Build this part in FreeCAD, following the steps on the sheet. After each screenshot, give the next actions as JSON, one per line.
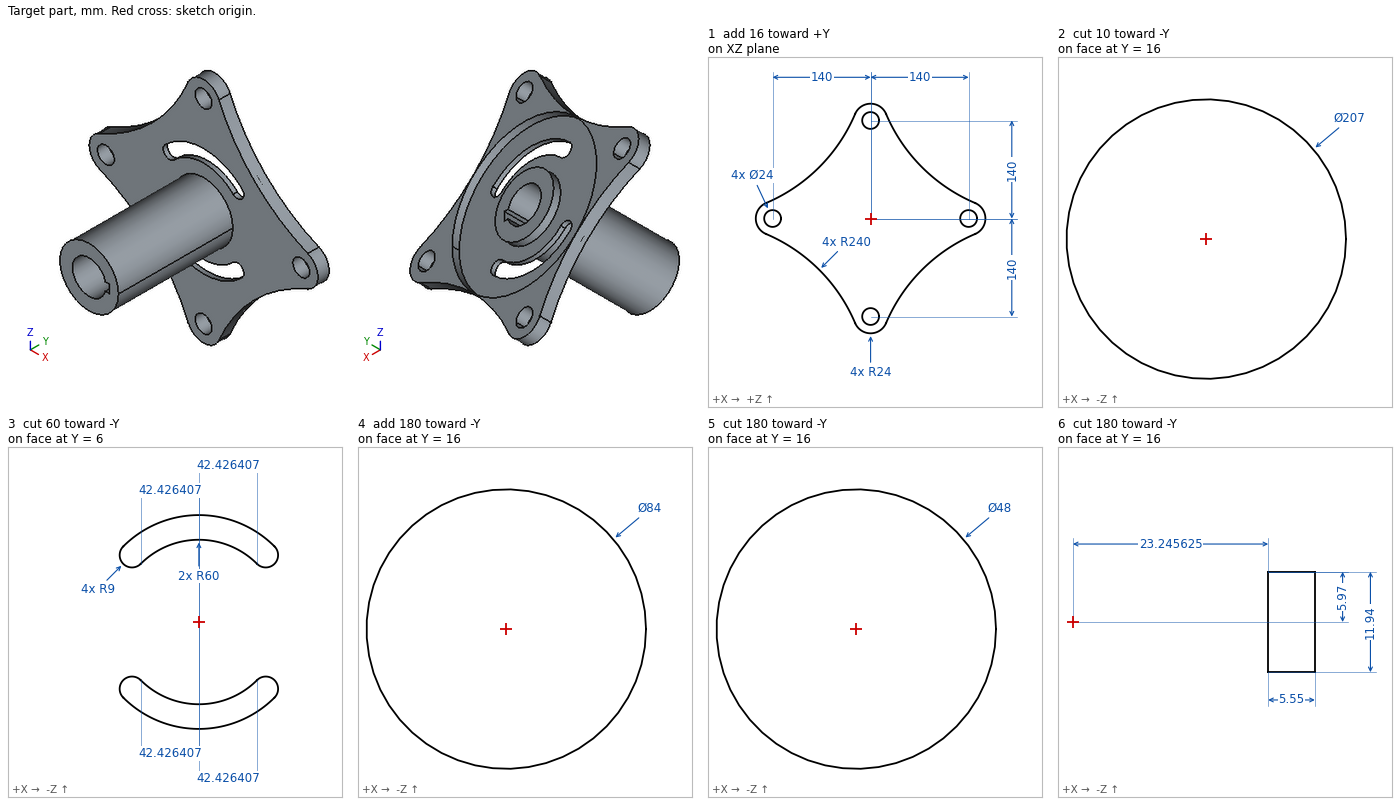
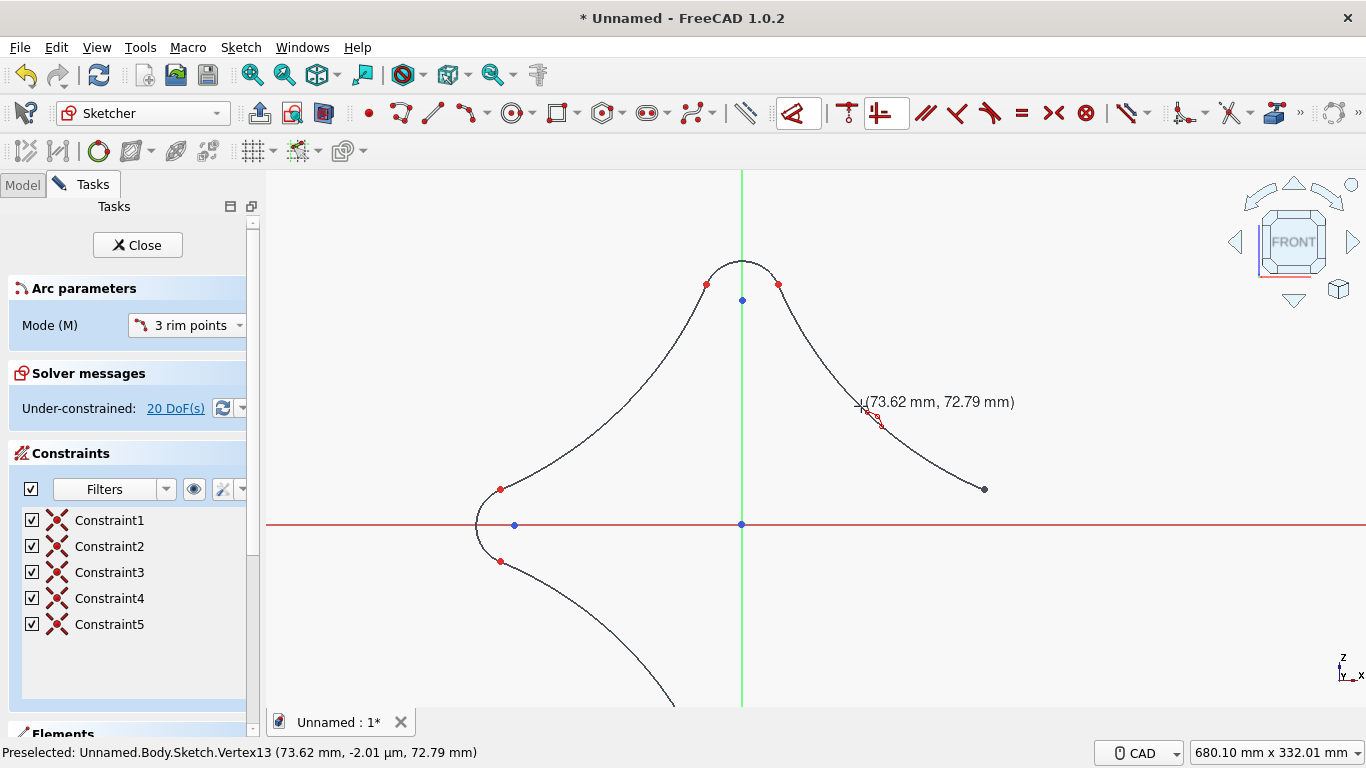
{"action": "left_click", "coordinate": [984, 490]}
{"action": "left_click", "coordinate": [984, 560]}
{"action": "left_click", "coordinate": [1003, 542]}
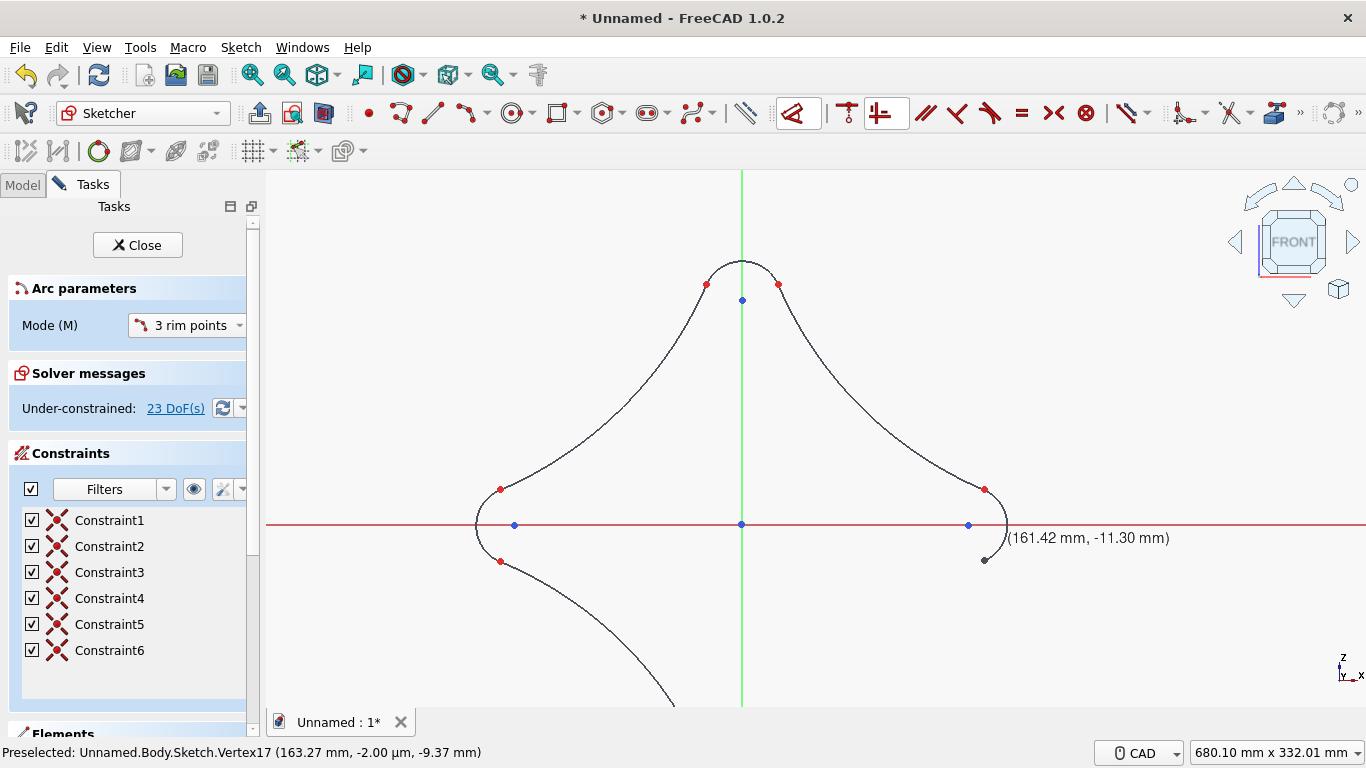
{"action": "left_click", "coordinate": [984, 561]}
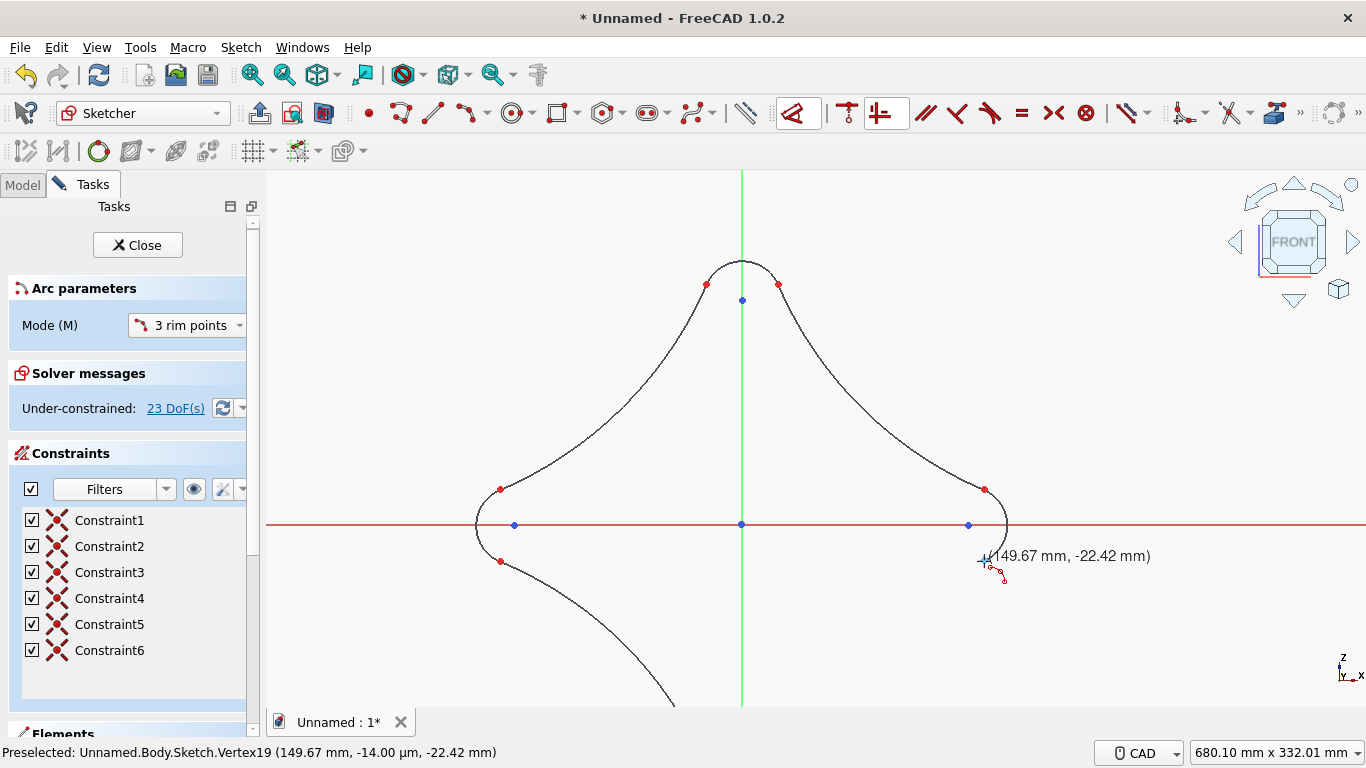
{"action": "scroll", "coordinate": [759, 263], "scroll_direction": "down", "scroll_amount": 2}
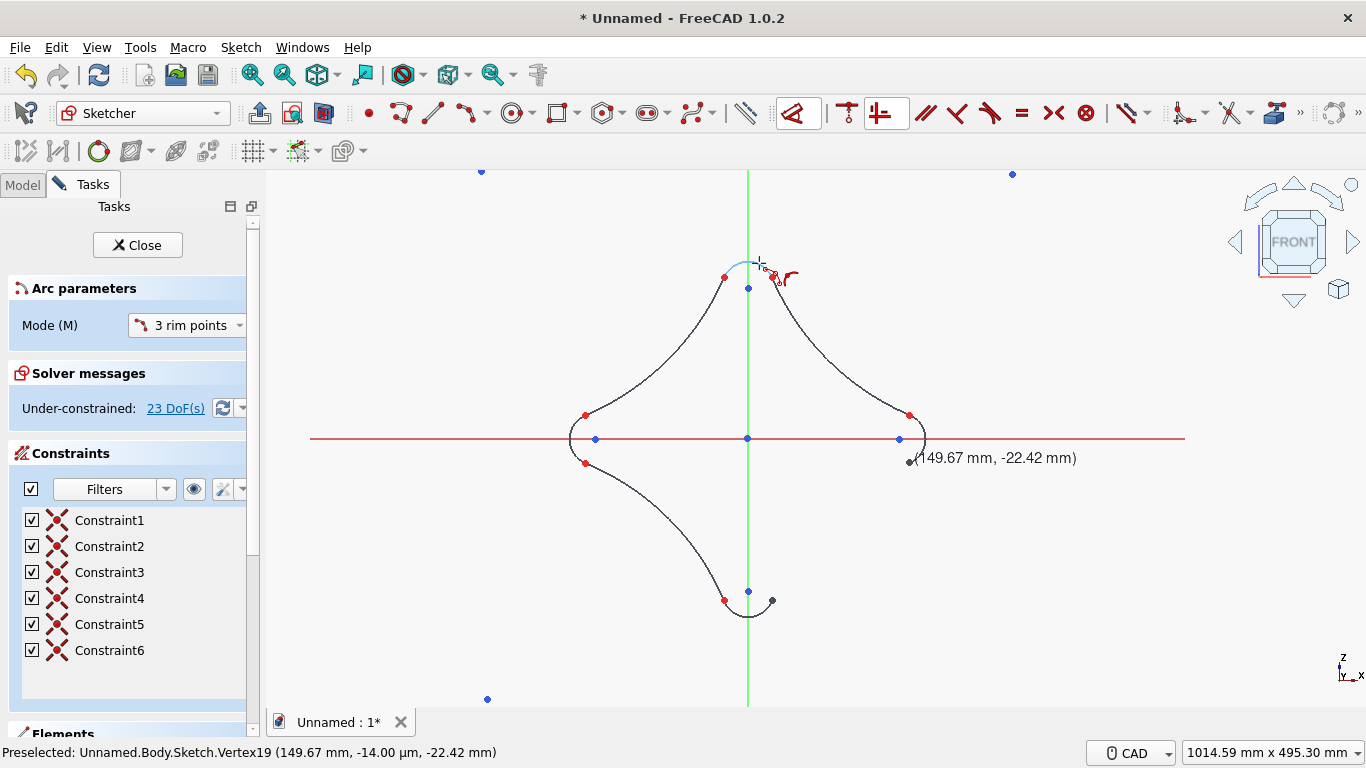
{"action": "left_click", "coordinate": [772, 601]}
{"action": "left_click", "coordinate": [827, 518]}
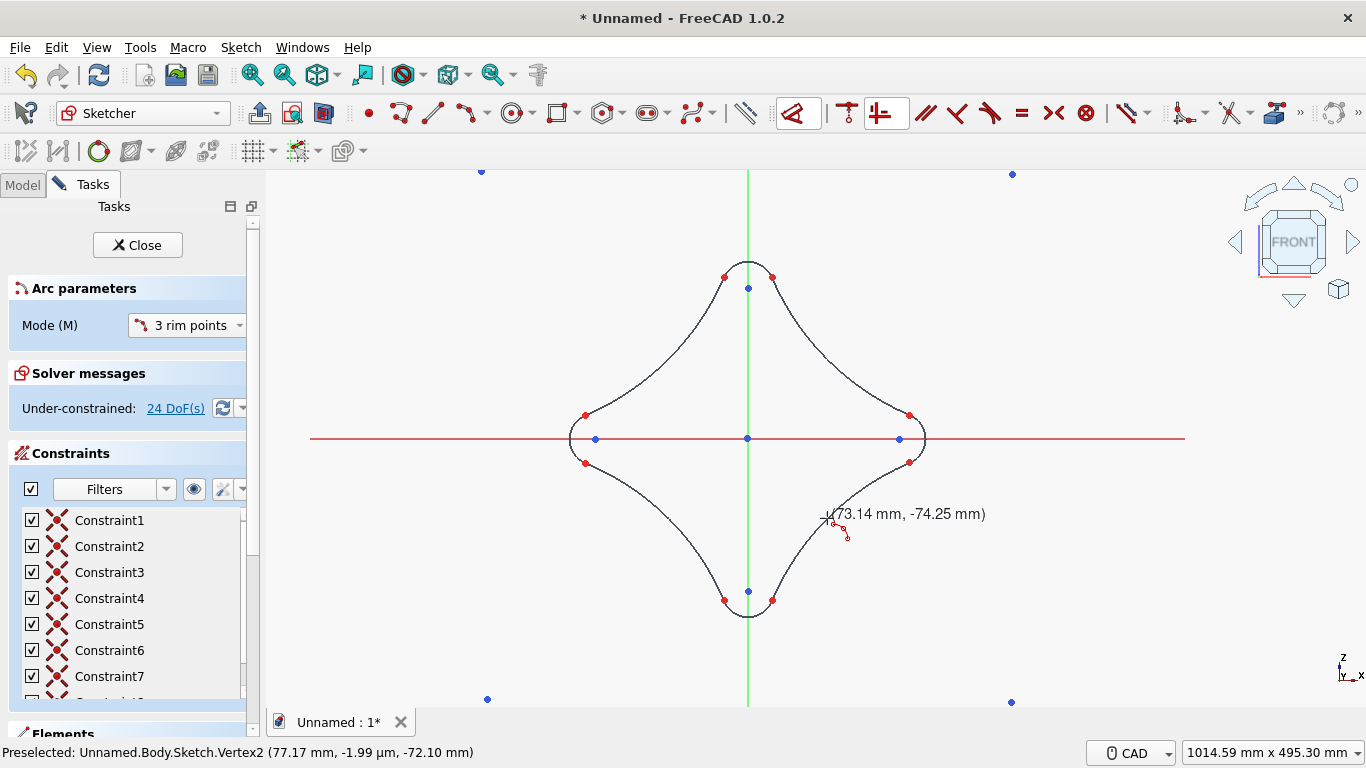
{"action": "left_click", "coordinate": [512, 114]}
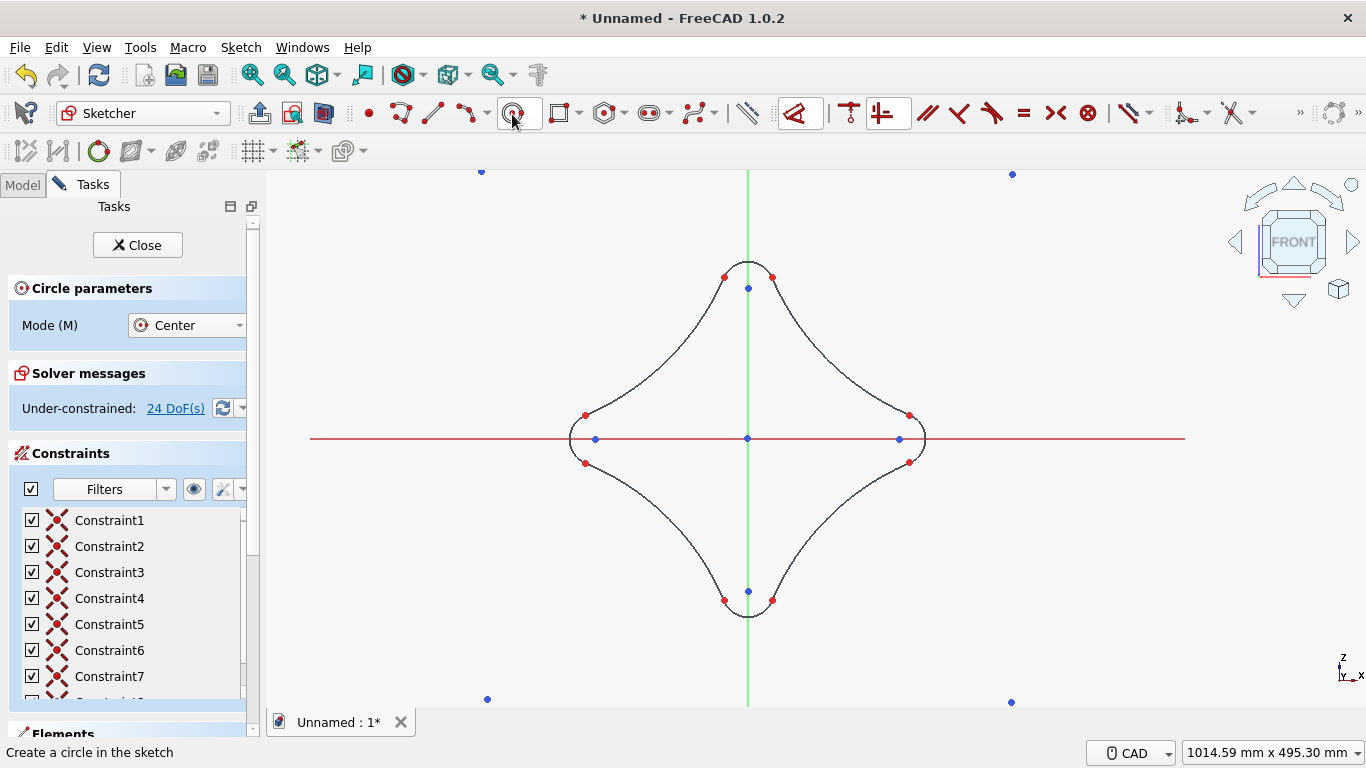
{"action": "scroll", "coordinate": [748, 287], "scroll_direction": "up", "scroll_amount": 3}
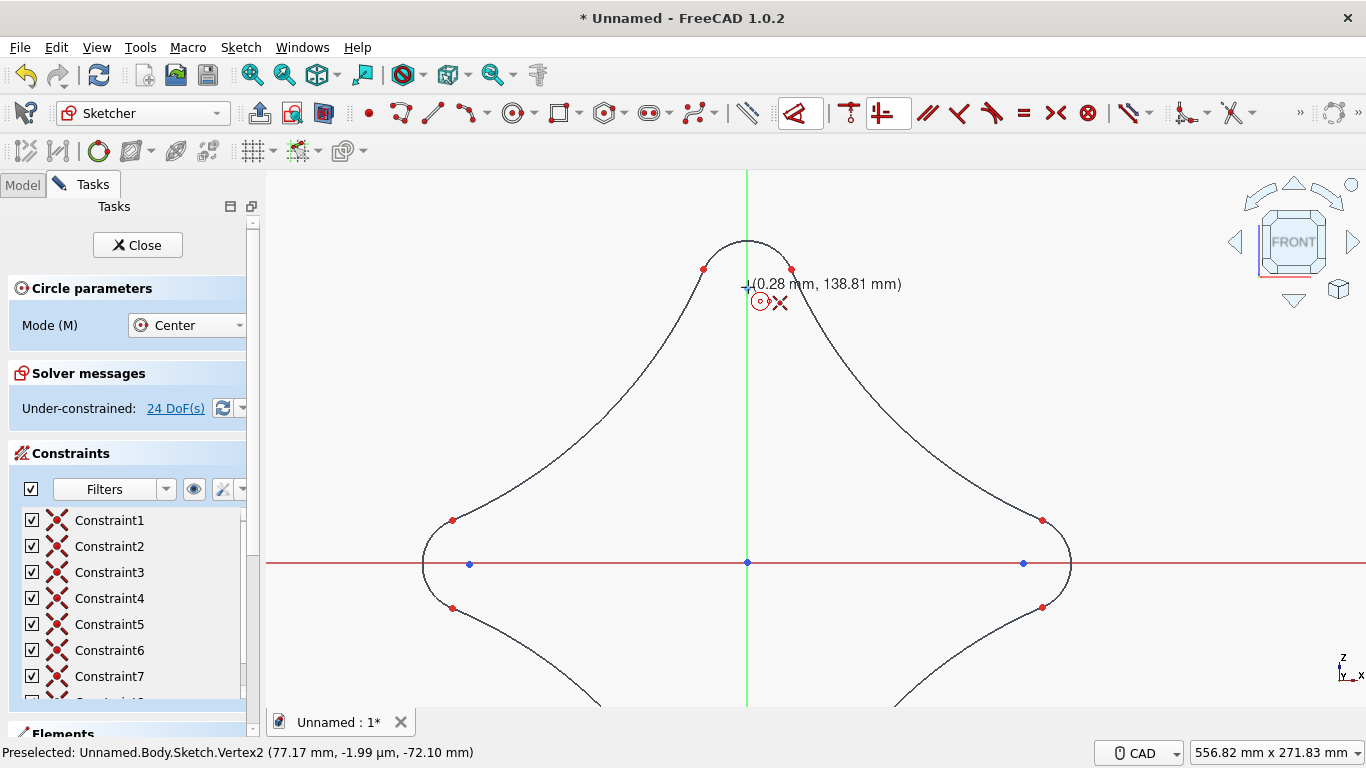
{"action": "left_click", "coordinate": [747, 286]}
{"action": "left_click", "coordinate": [764, 270]}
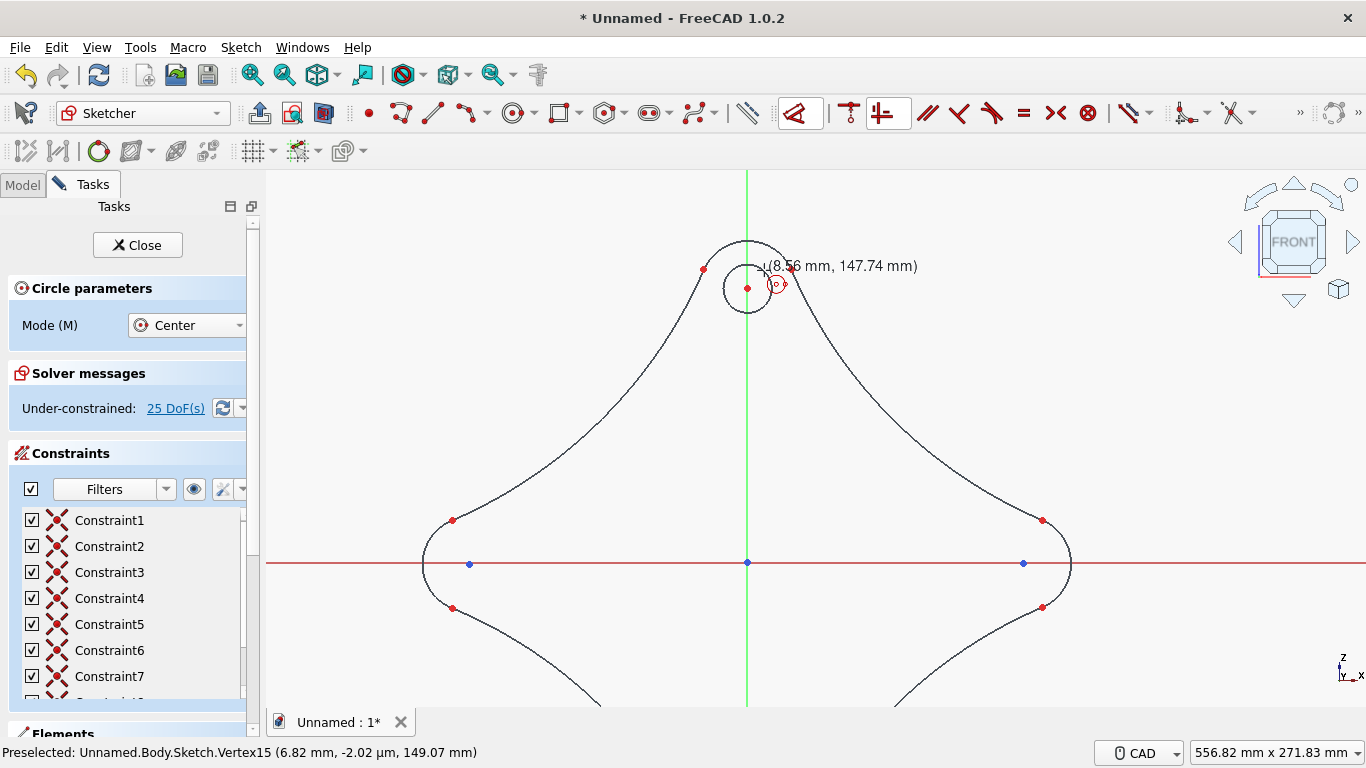
{"action": "left_click", "coordinate": [471, 563]}
{"action": "left_click", "coordinate": [487, 546]}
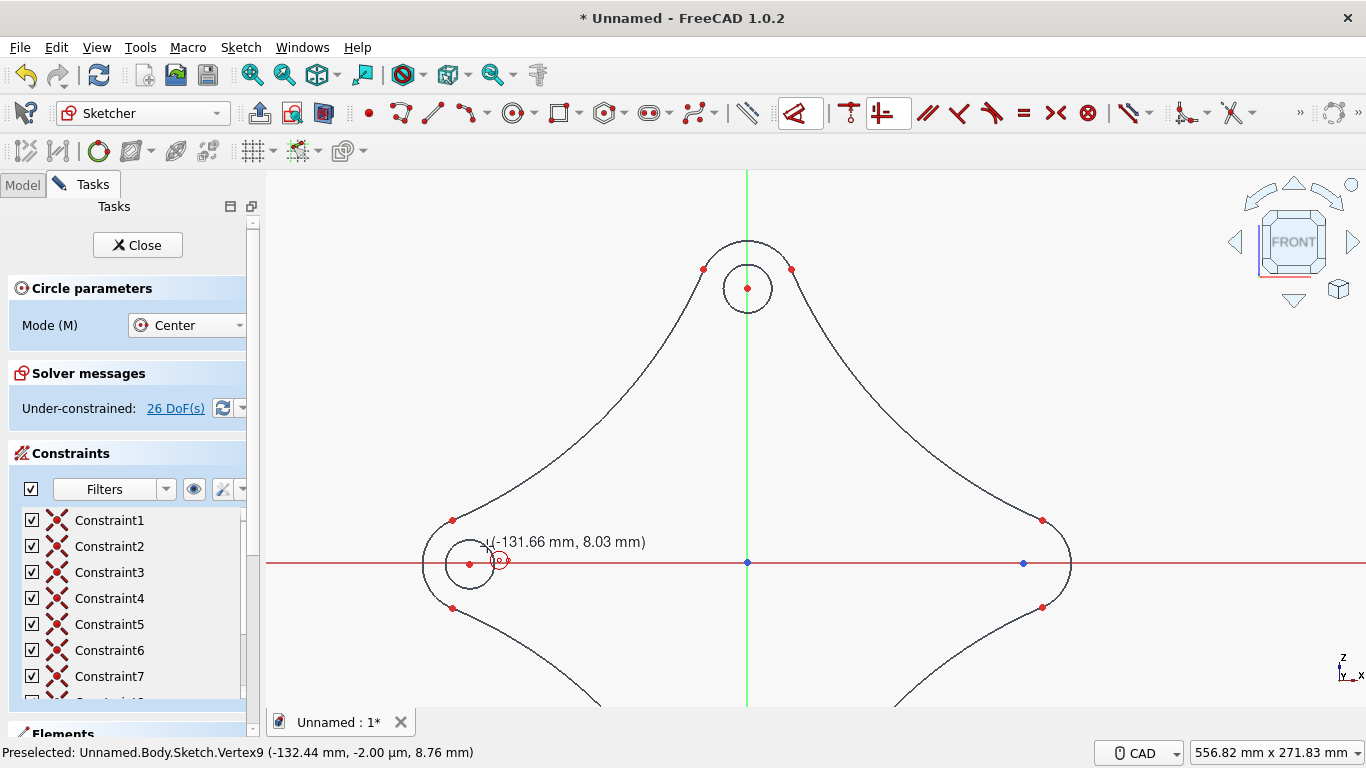
{"action": "left_click", "coordinate": [1024, 563]}
{"action": "left_click", "coordinate": [1040, 546]}